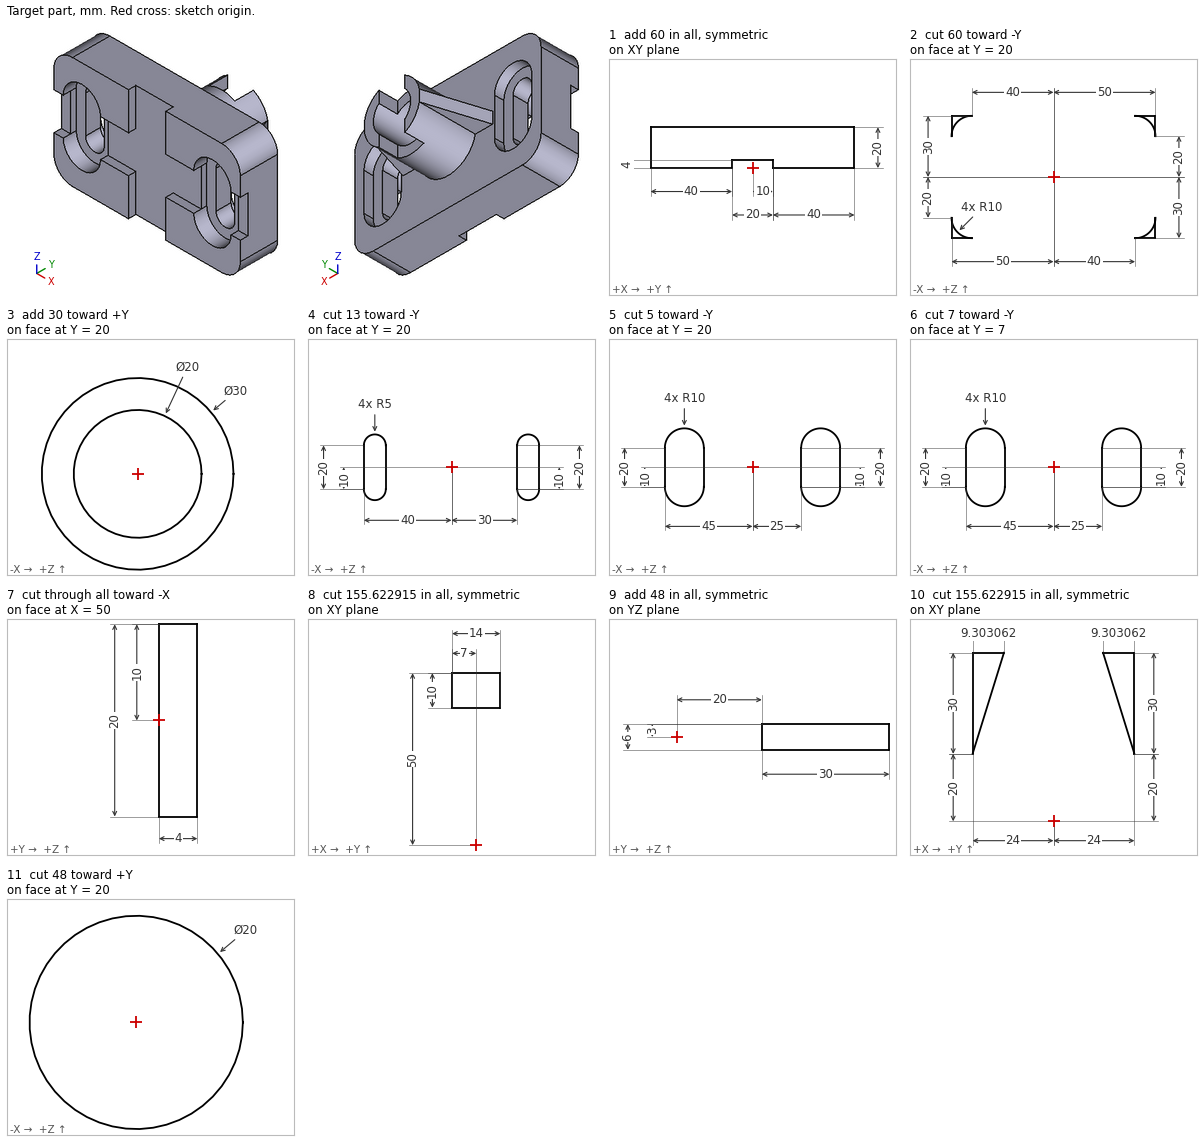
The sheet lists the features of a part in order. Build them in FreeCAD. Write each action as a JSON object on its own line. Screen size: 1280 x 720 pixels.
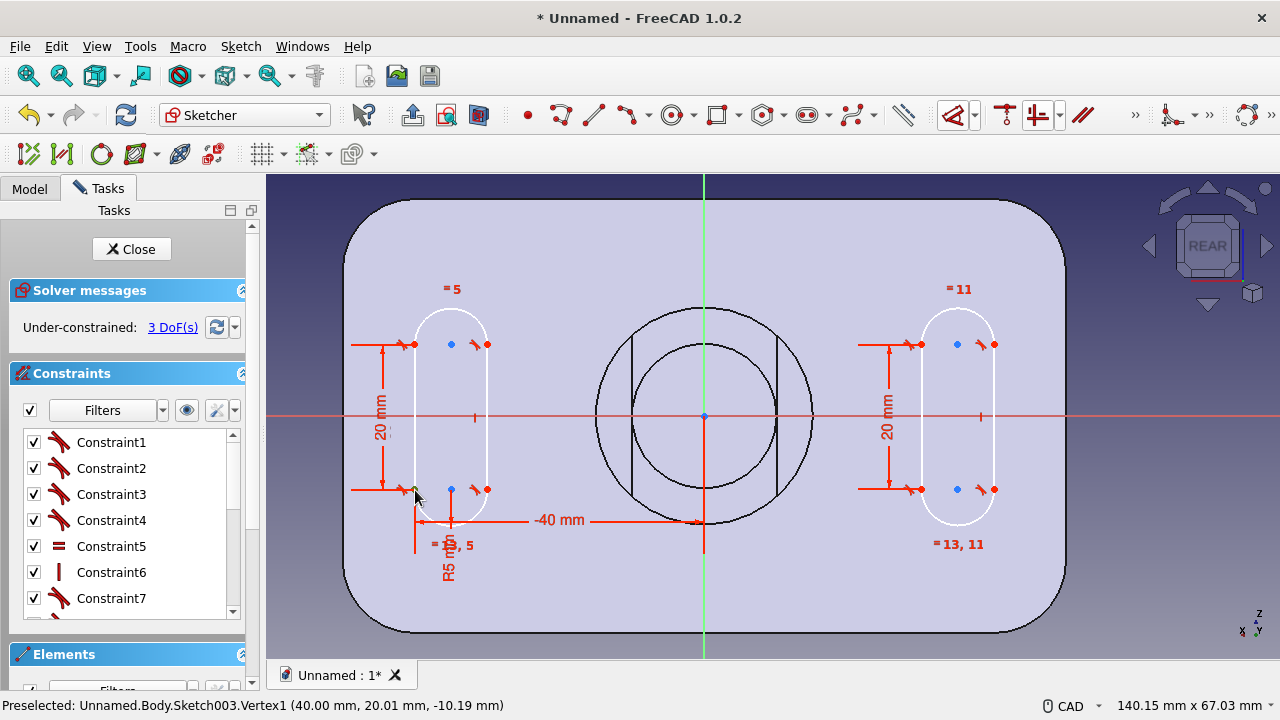
{"action": "key", "text": "i"}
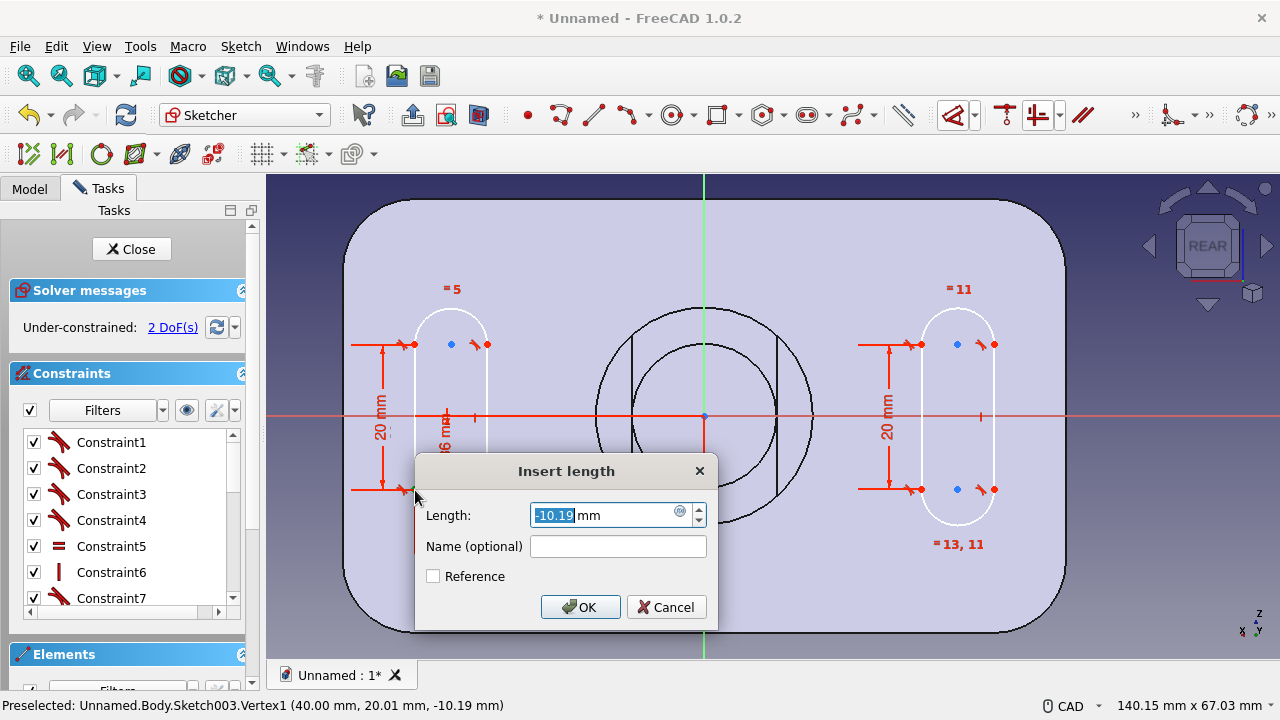
{"action": "type", "text": "-10"}
{"action": "key", "text": "Return"}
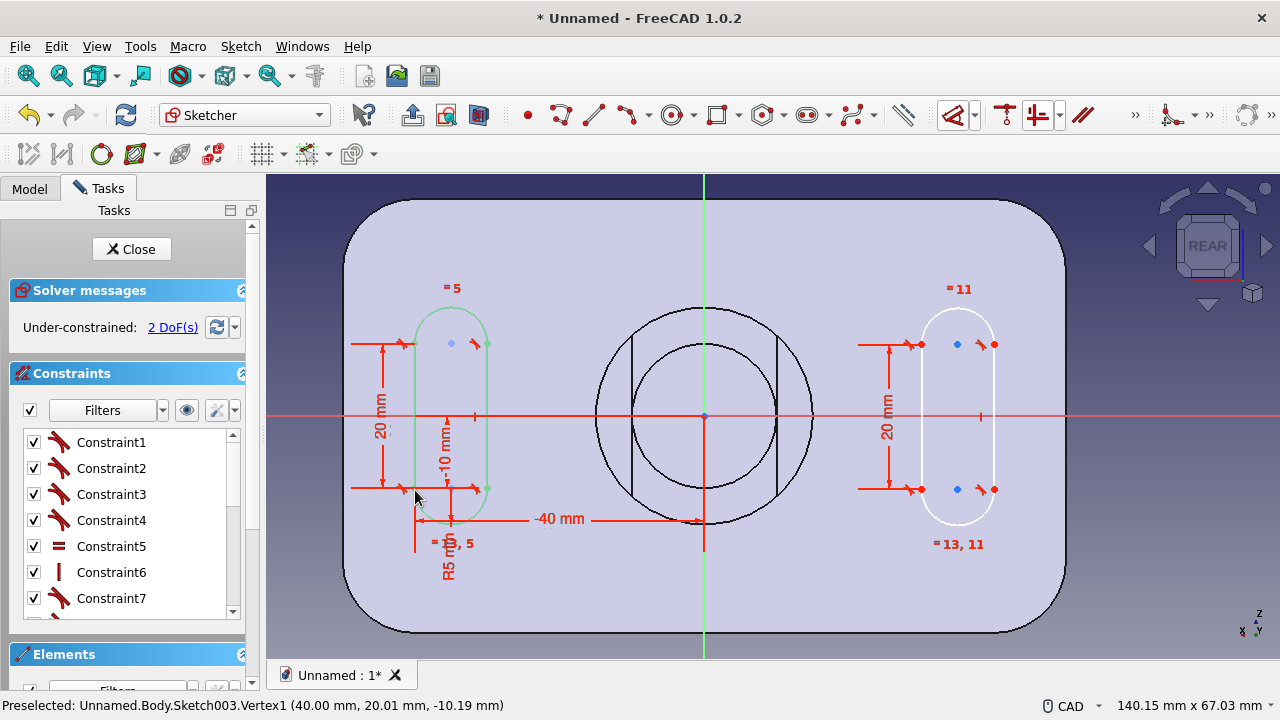
{"action": "left_click", "coordinate": [922, 489]}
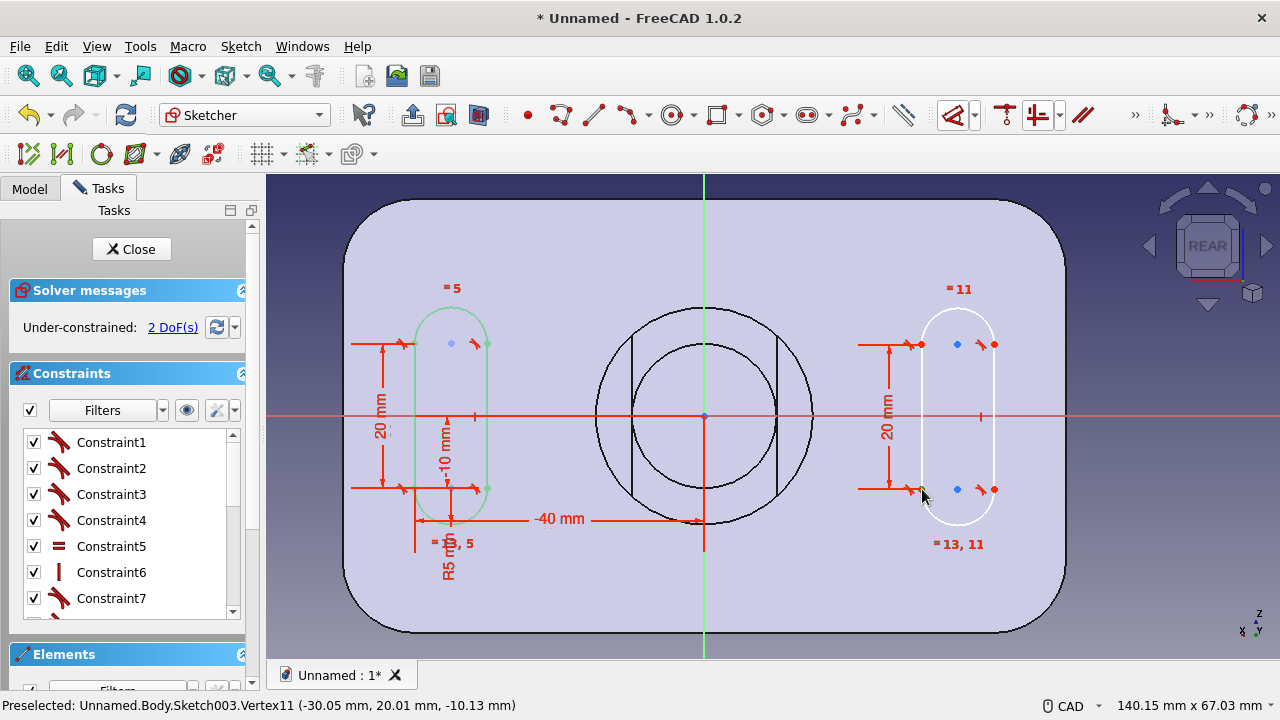
{"action": "key", "text": "l"}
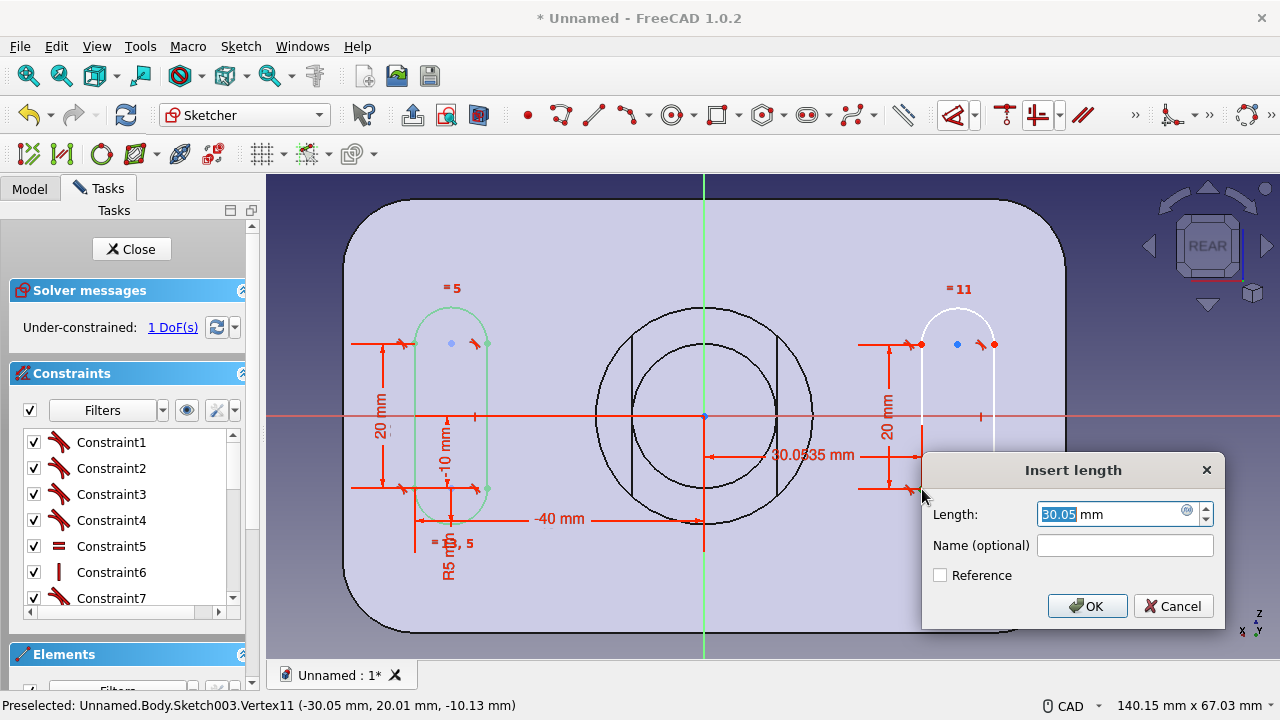
{"action": "type", "text": "30"}
{"action": "key", "text": "Return"}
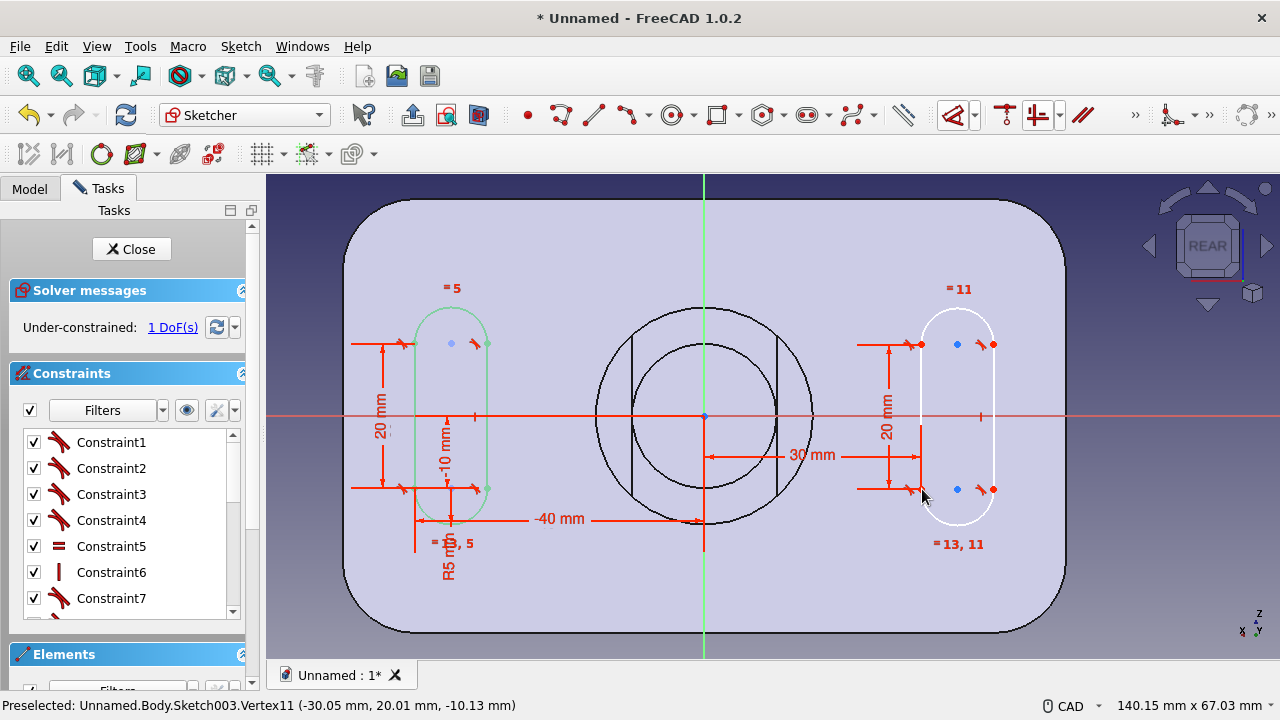
{"action": "left_click", "coordinate": [921, 489]}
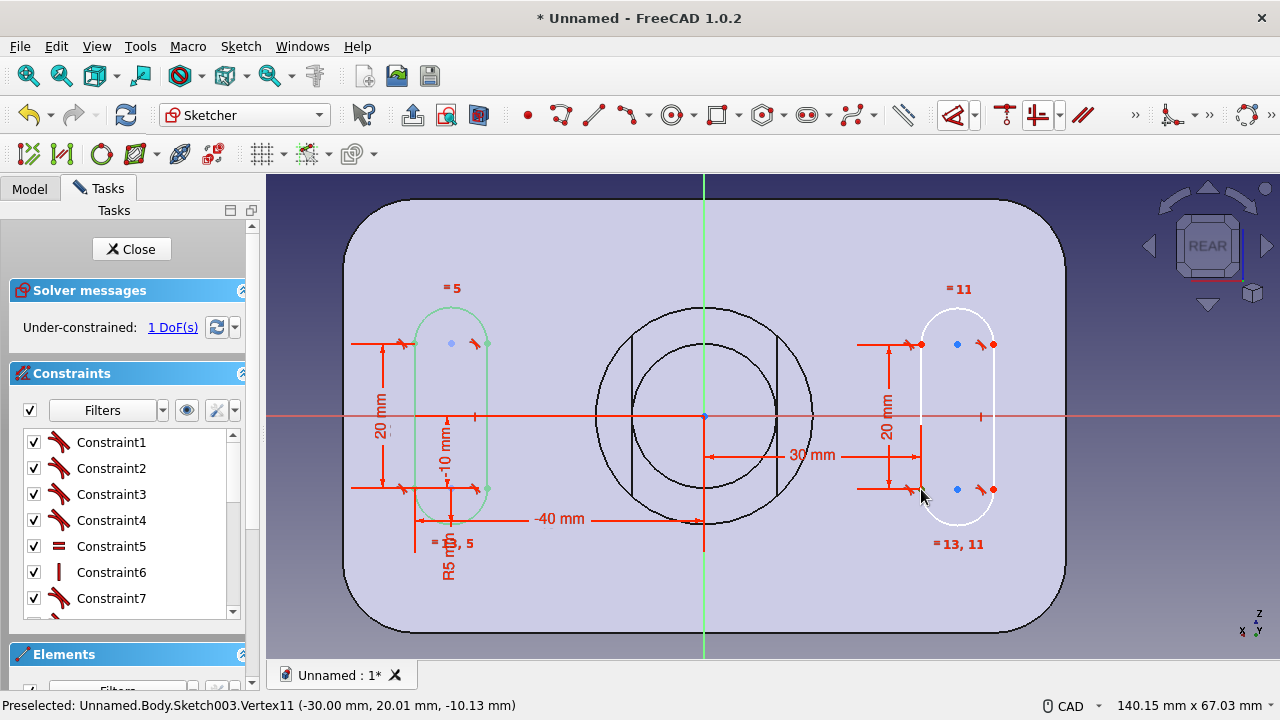
{"action": "key", "text": "i"}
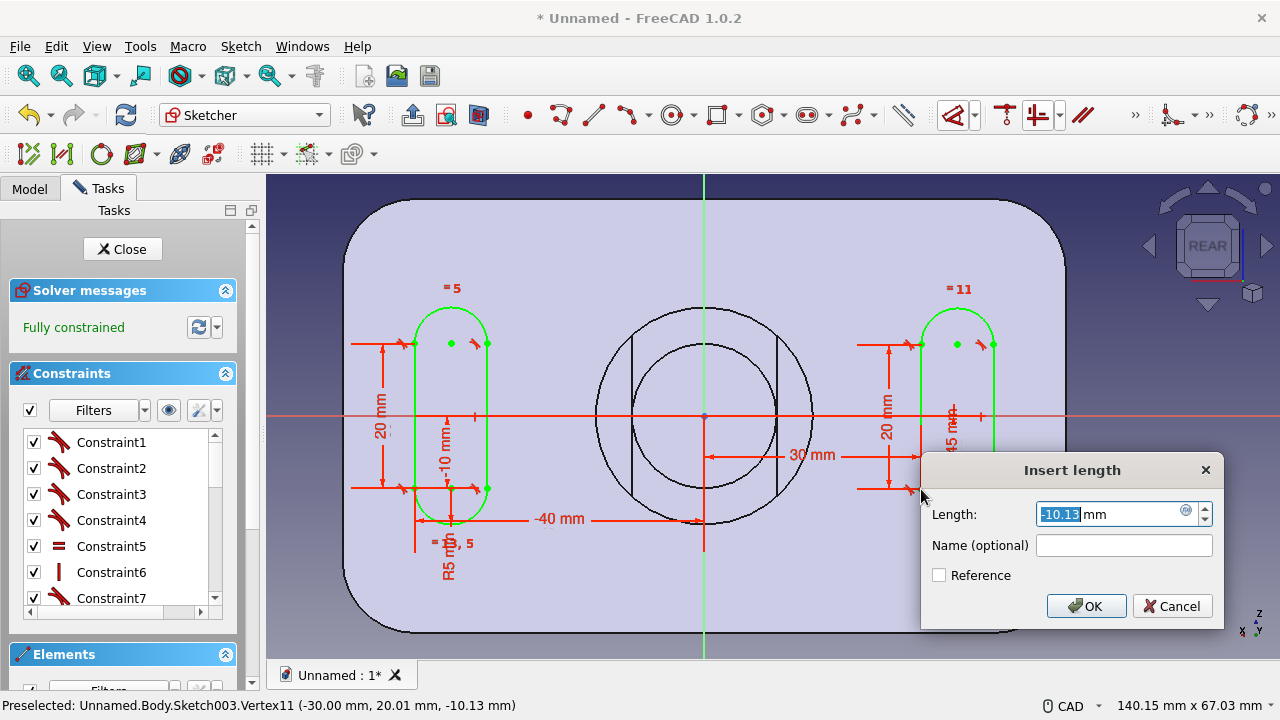
{"action": "type", "text": "-10"}
{"action": "key", "text": "Return"}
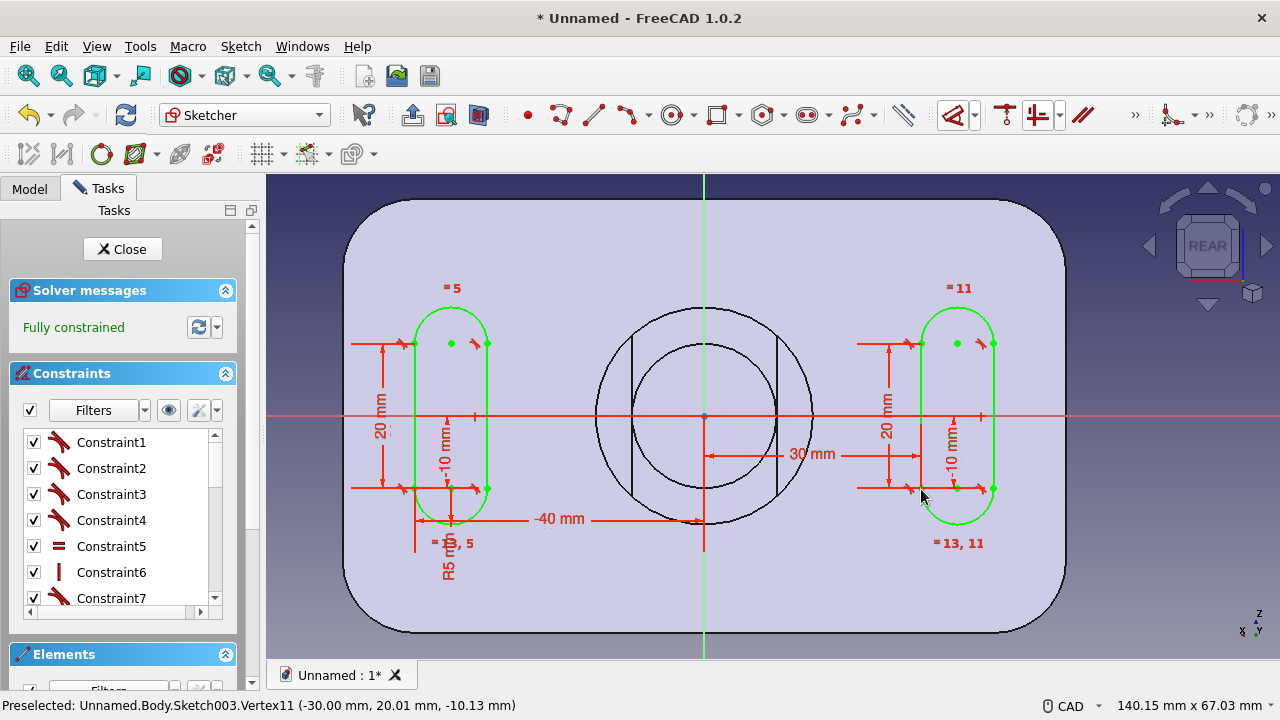
{"action": "left_click", "coordinate": [123, 249]}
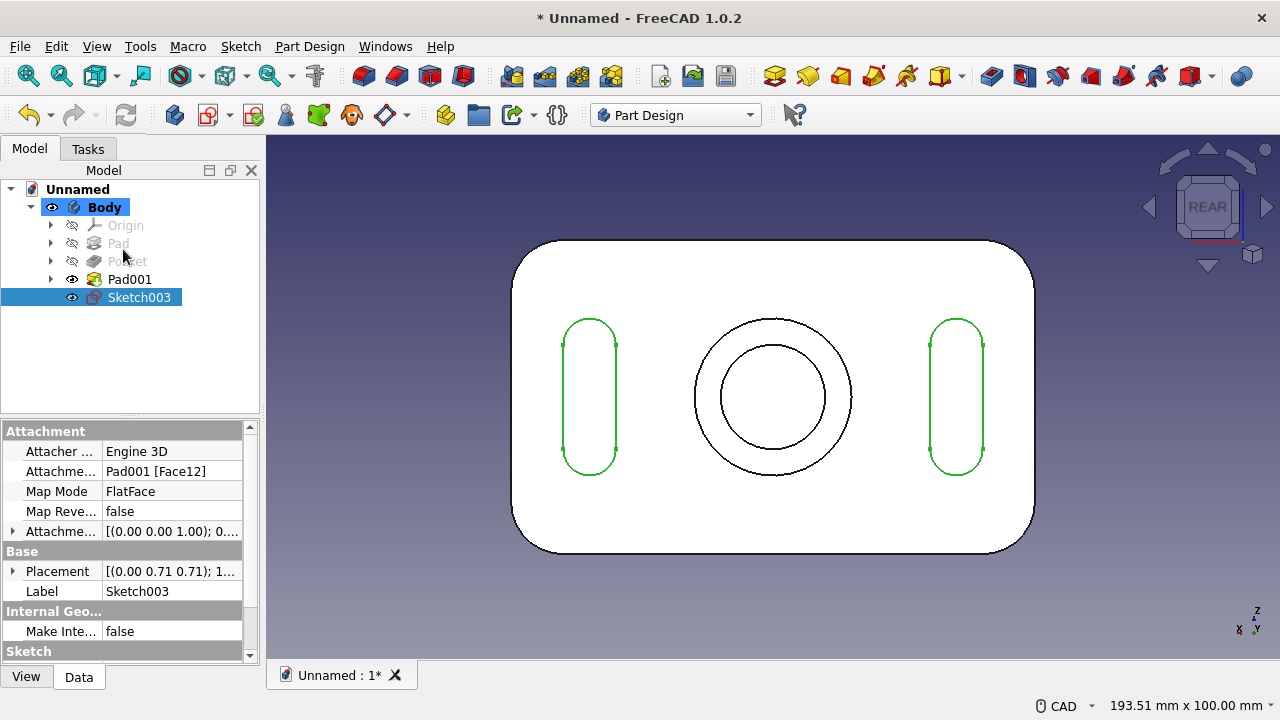
{"action": "left_click", "coordinate": [992, 76]}